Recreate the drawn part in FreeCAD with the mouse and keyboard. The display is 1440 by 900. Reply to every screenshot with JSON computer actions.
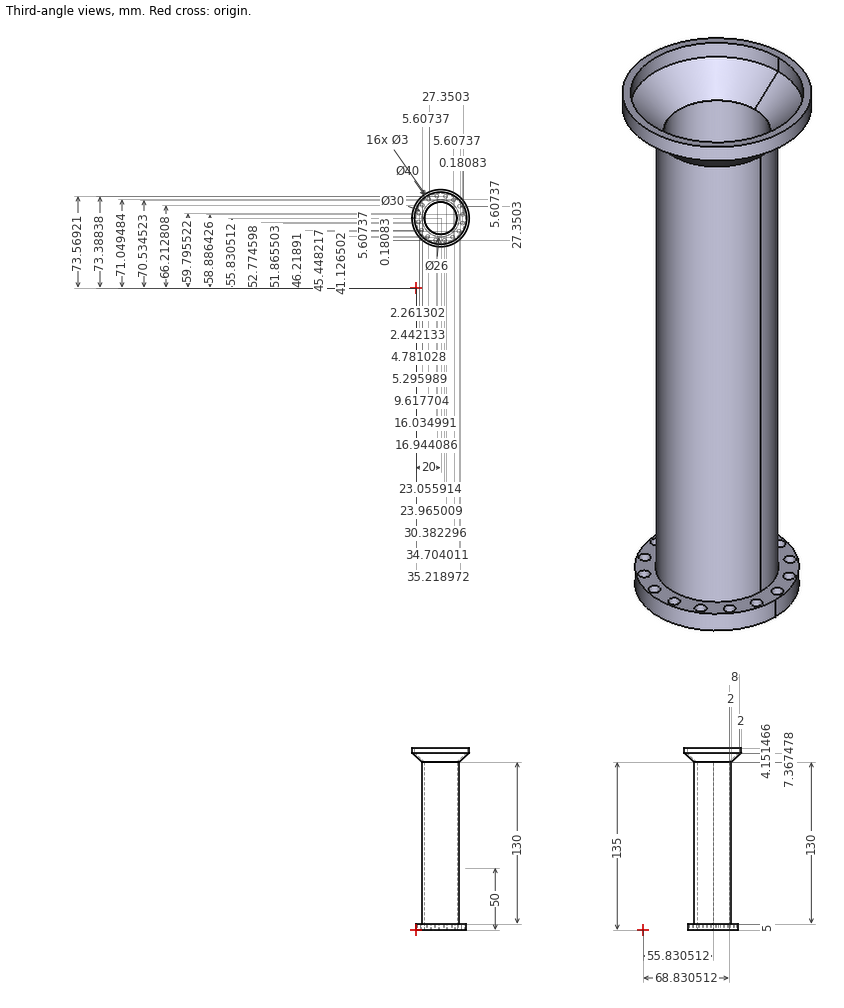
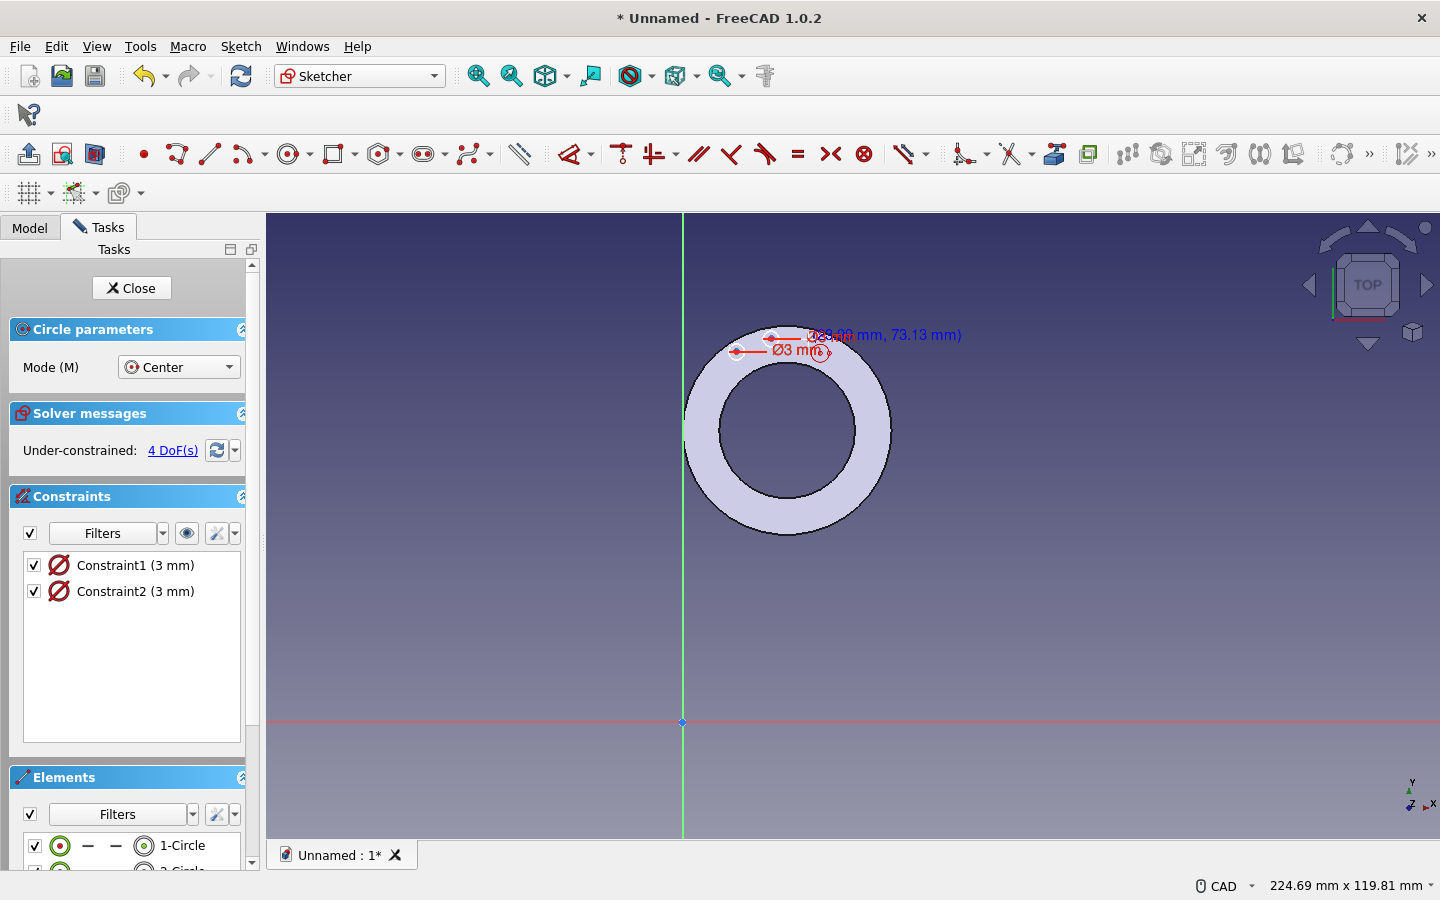
{"action": "left_click", "coordinate": [808, 339]}
{"action": "mouse_move", "coordinate": [813, 333]}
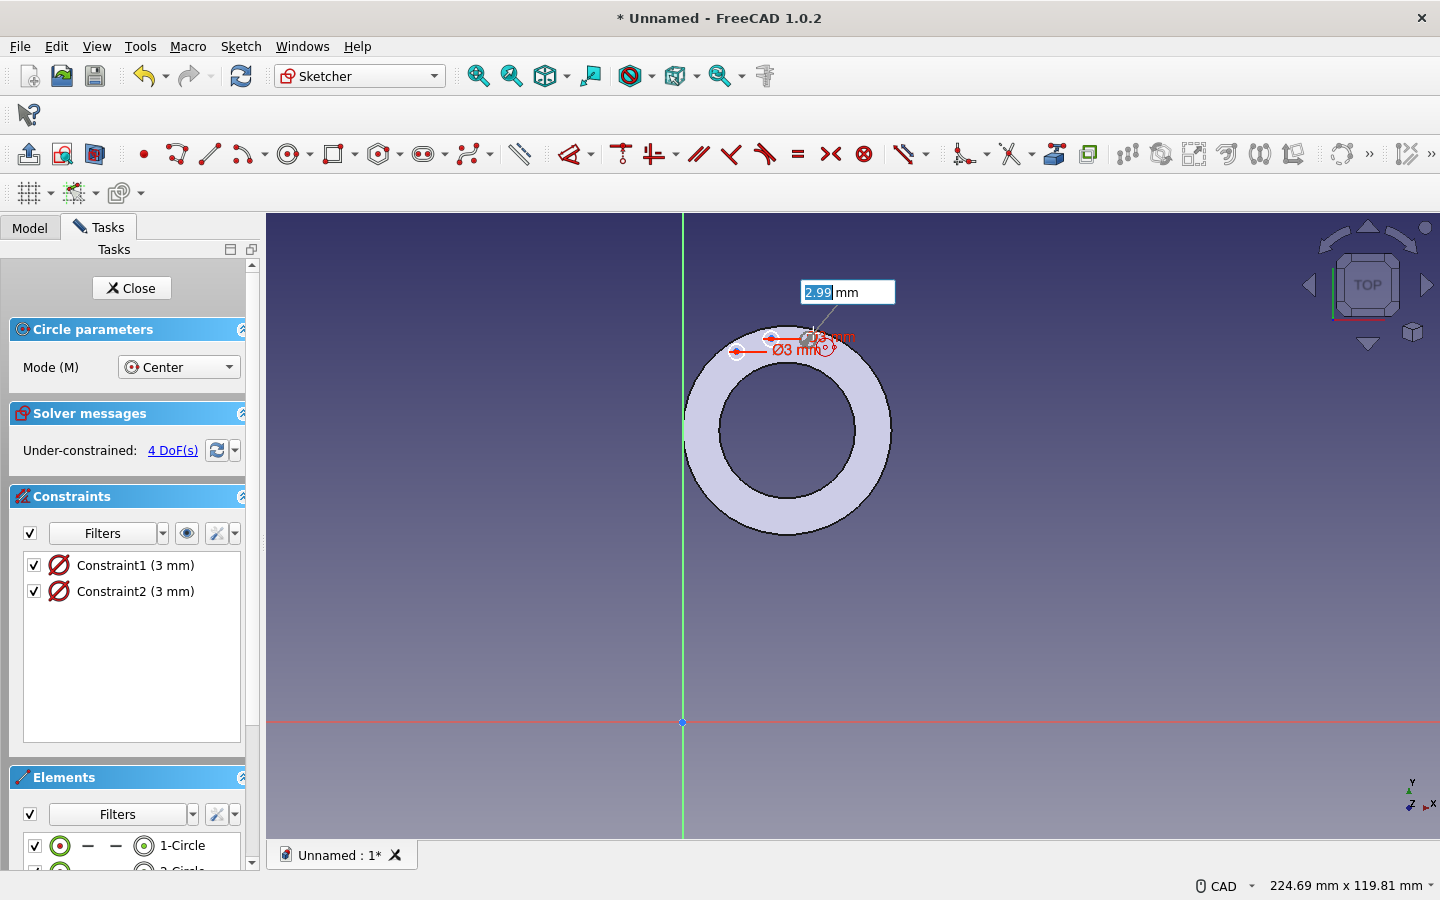
{"action": "type", "text": "3"}
{"action": "key", "text": "Return"}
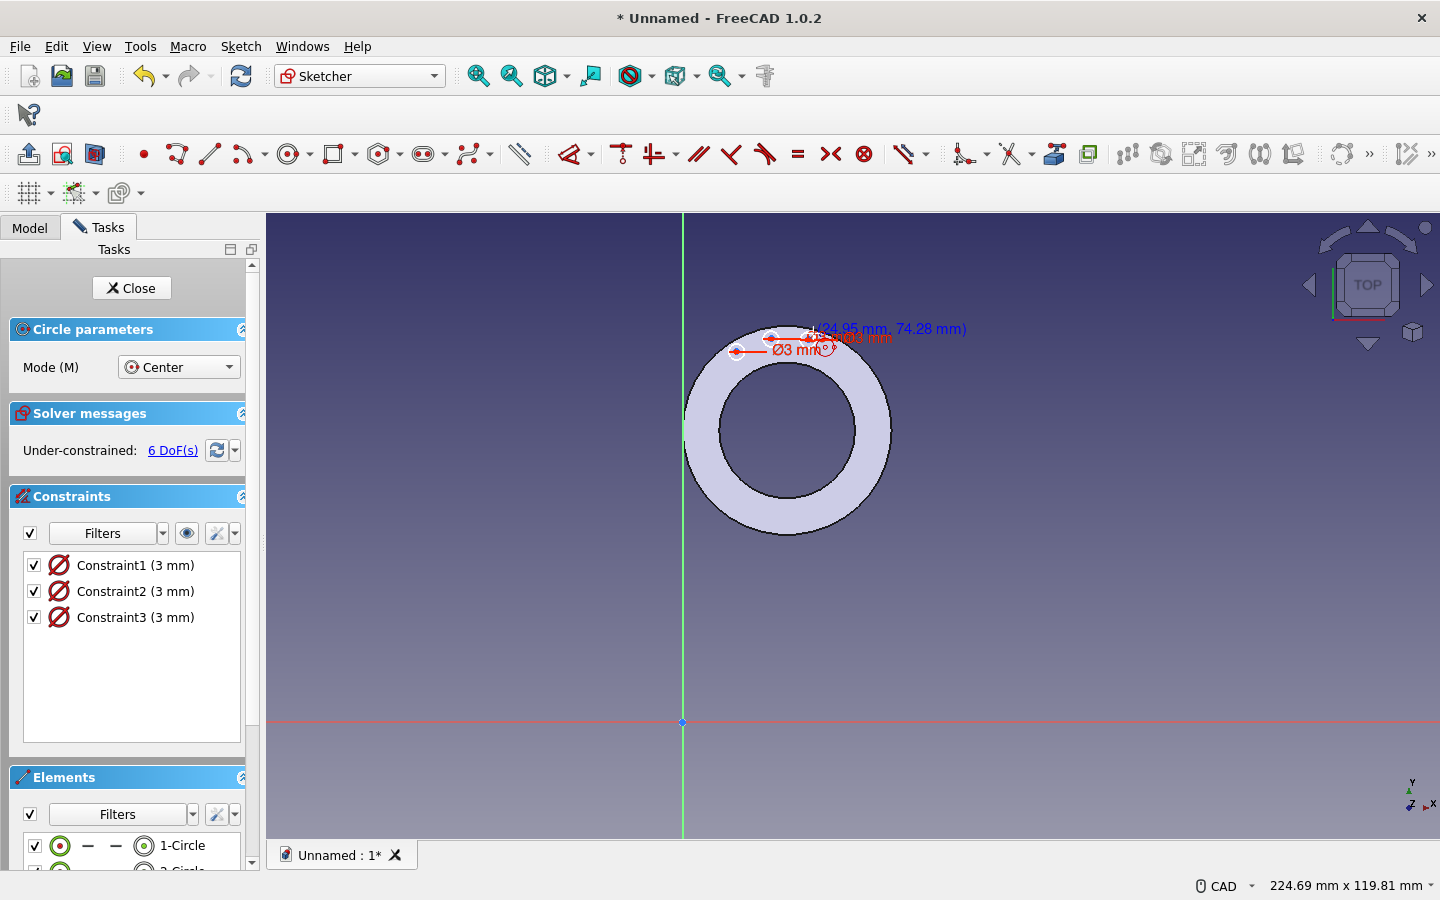
{"action": "scroll", "coordinate": [841, 354], "scroll_direction": "up", "scroll_amount": 6}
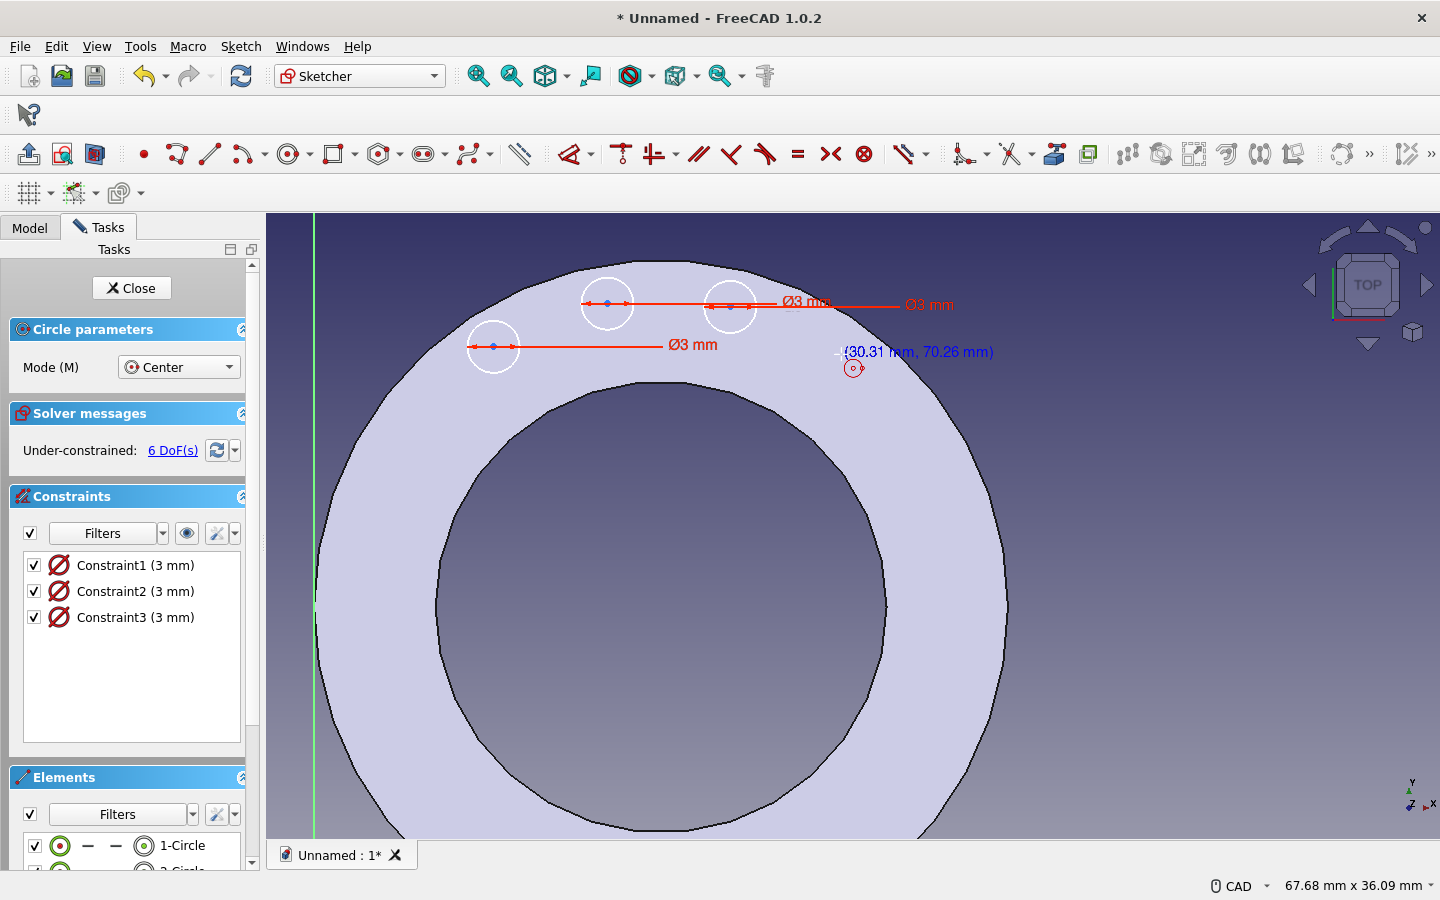
{"action": "scroll", "coordinate": [841, 354], "scroll_direction": "down", "scroll_amount": 6}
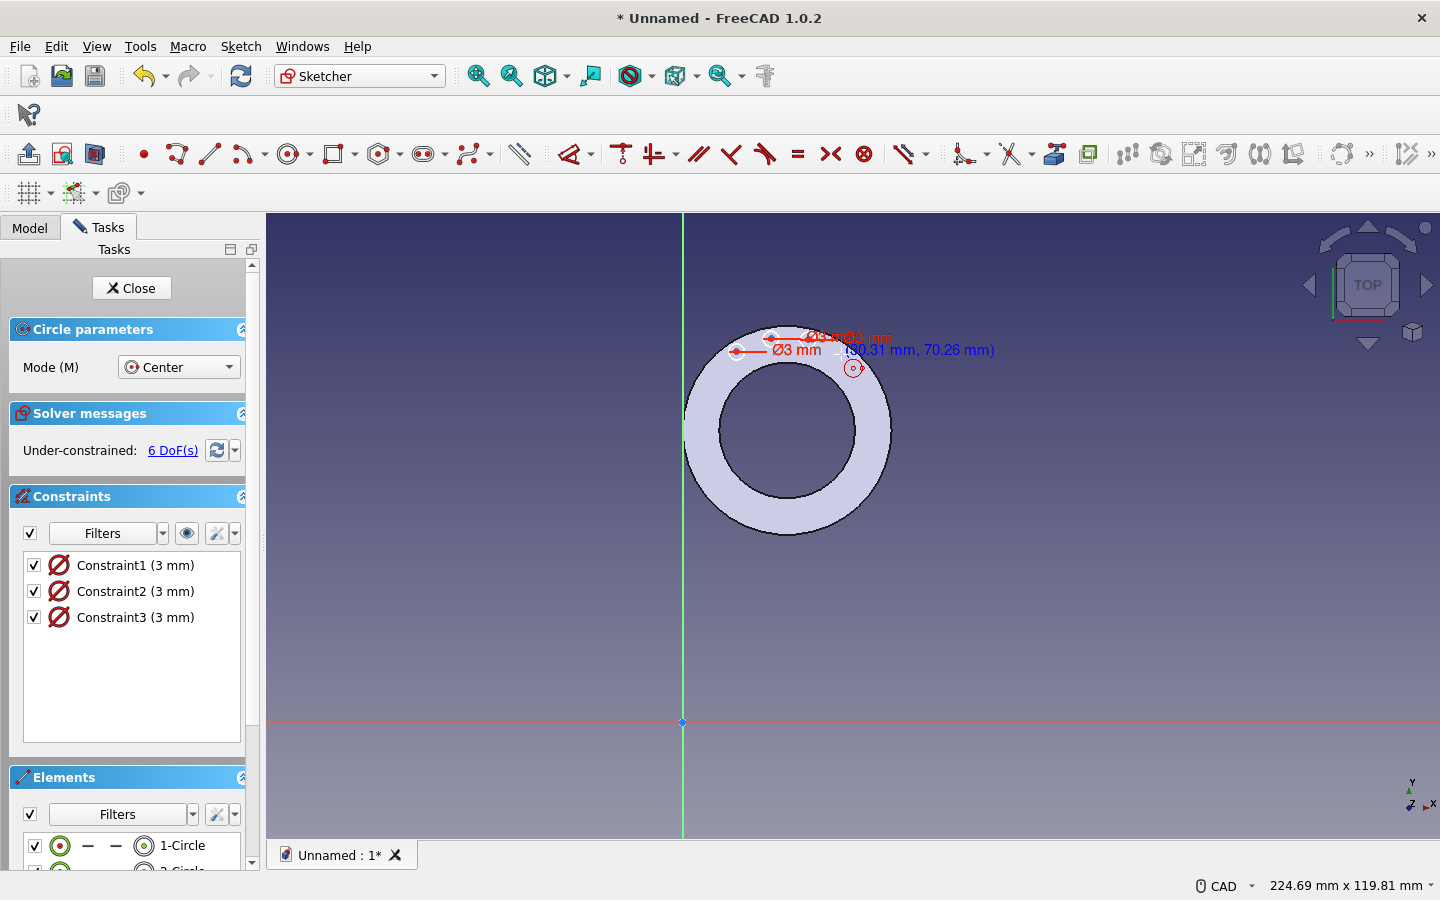
{"action": "left_click", "coordinate": [841, 354]}
{"action": "mouse_move", "coordinate": [847, 348]}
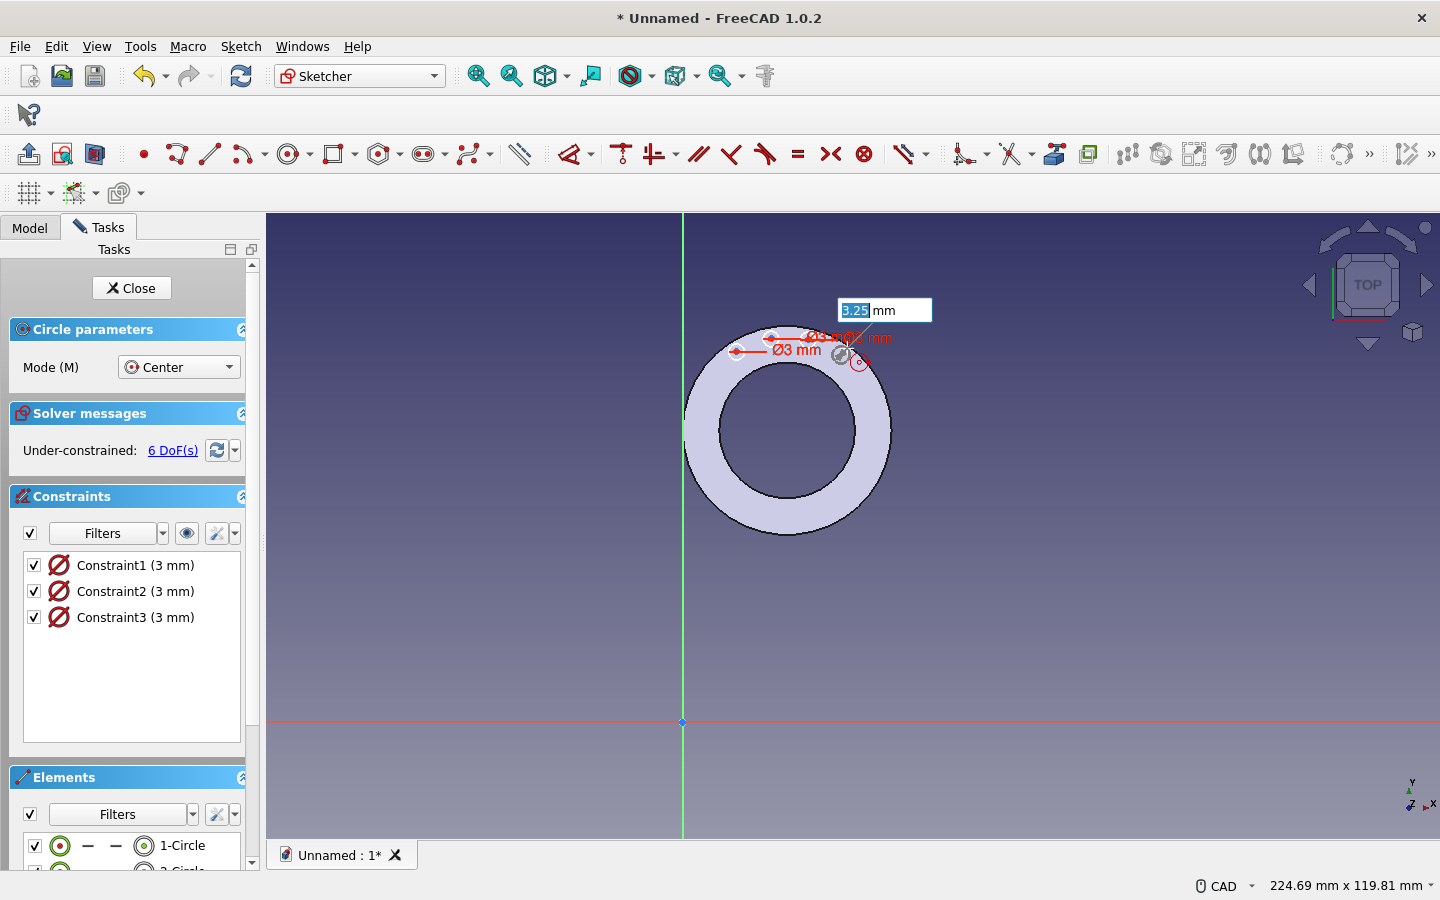
{"action": "type", "text": "3"}
{"action": "key", "text": "Return"}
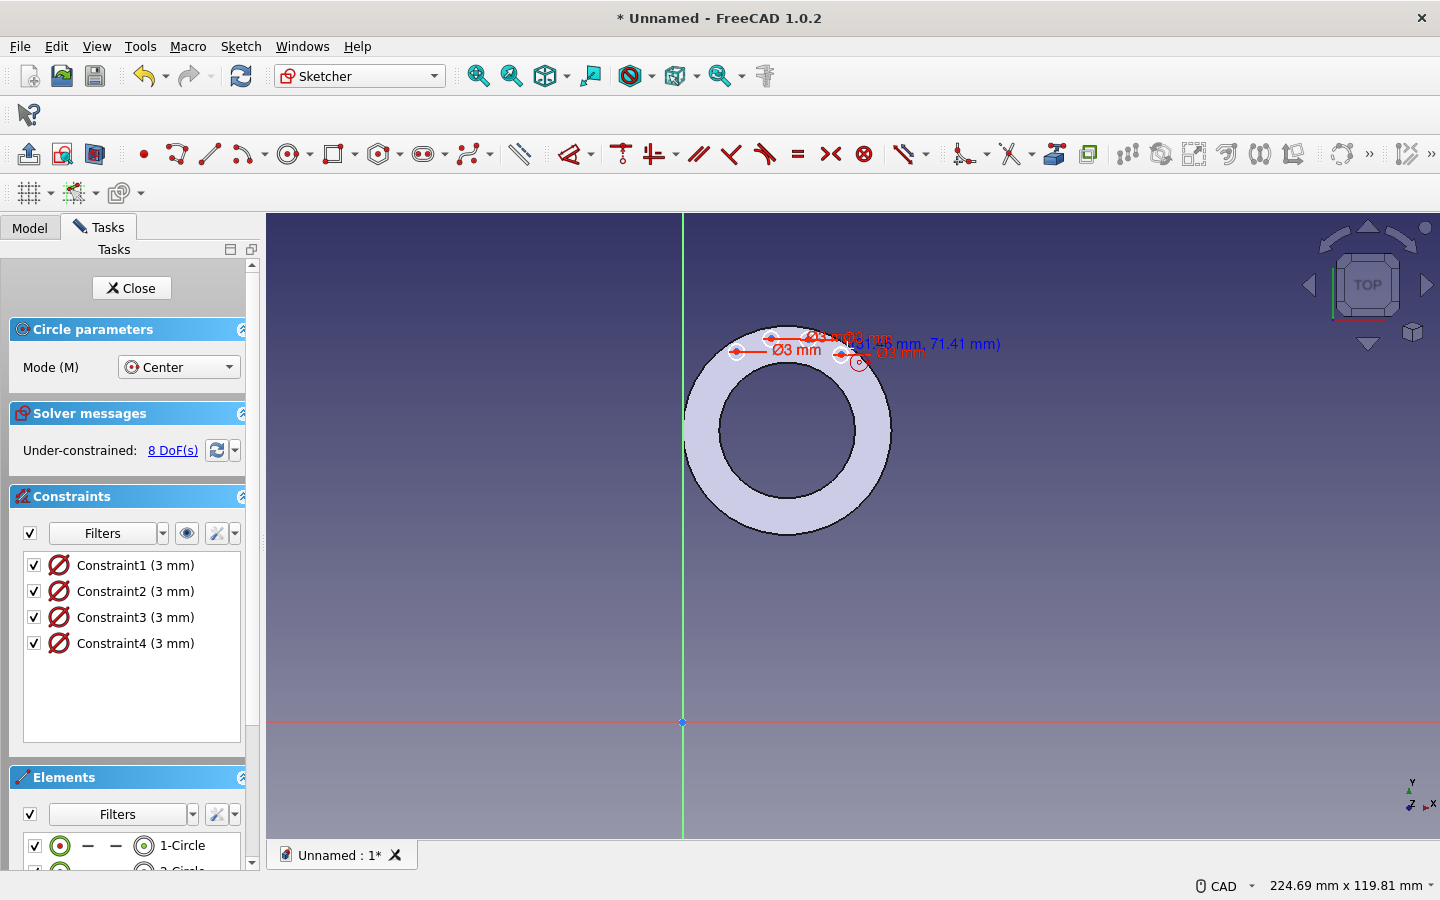
{"action": "scroll", "coordinate": [867, 380], "scroll_direction": "up", "scroll_amount": 6}